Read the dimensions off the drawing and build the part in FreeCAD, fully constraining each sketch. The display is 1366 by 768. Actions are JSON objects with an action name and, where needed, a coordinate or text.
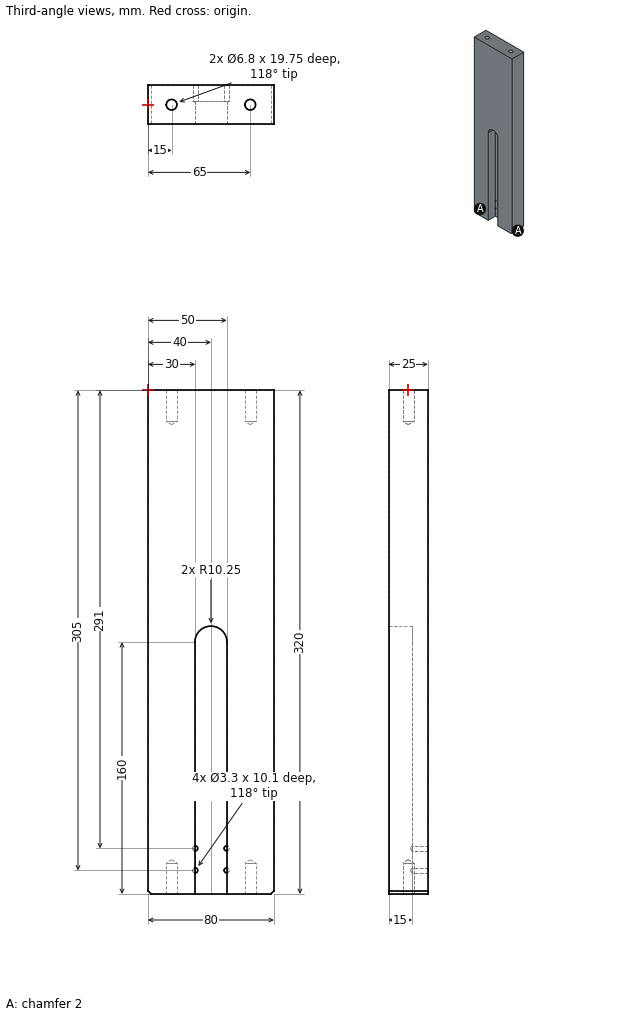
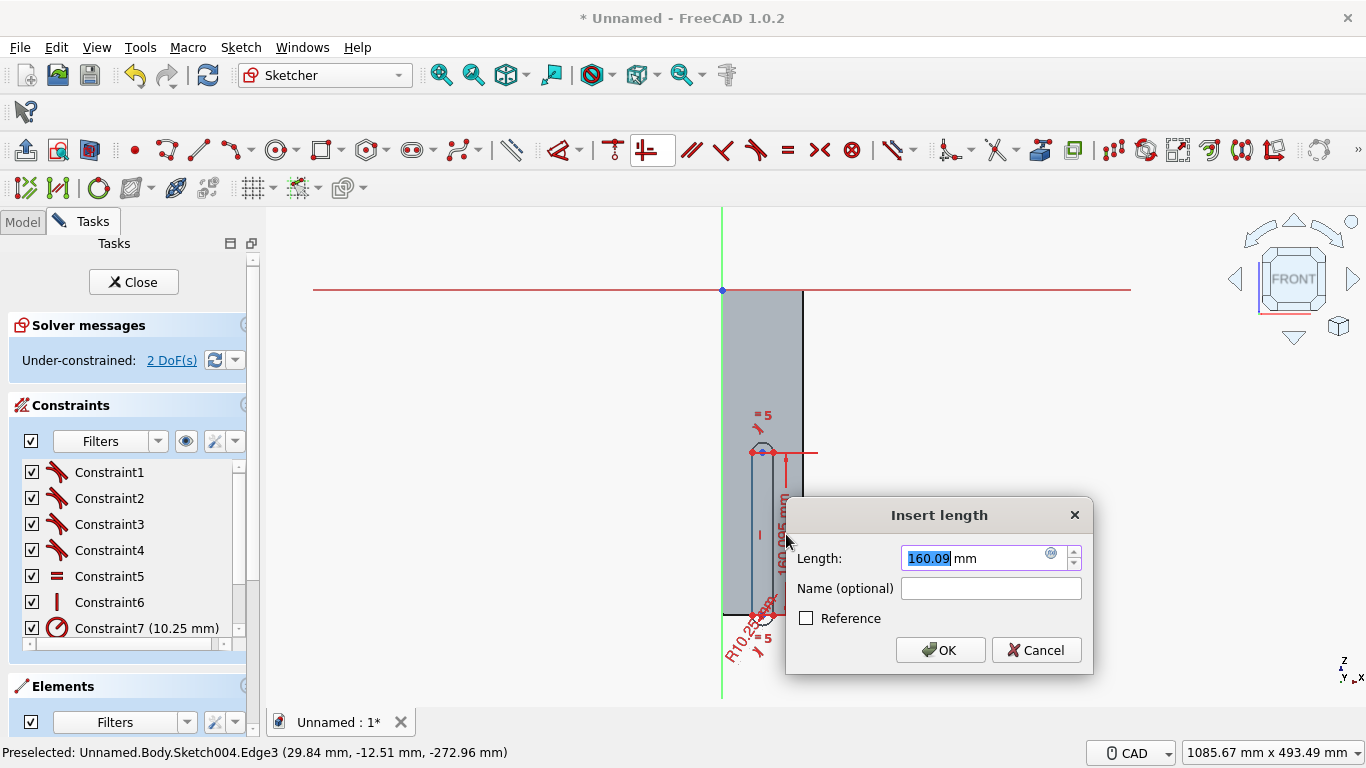
{"action": "type", "text": "160"}
{"action": "key", "text": "Return"}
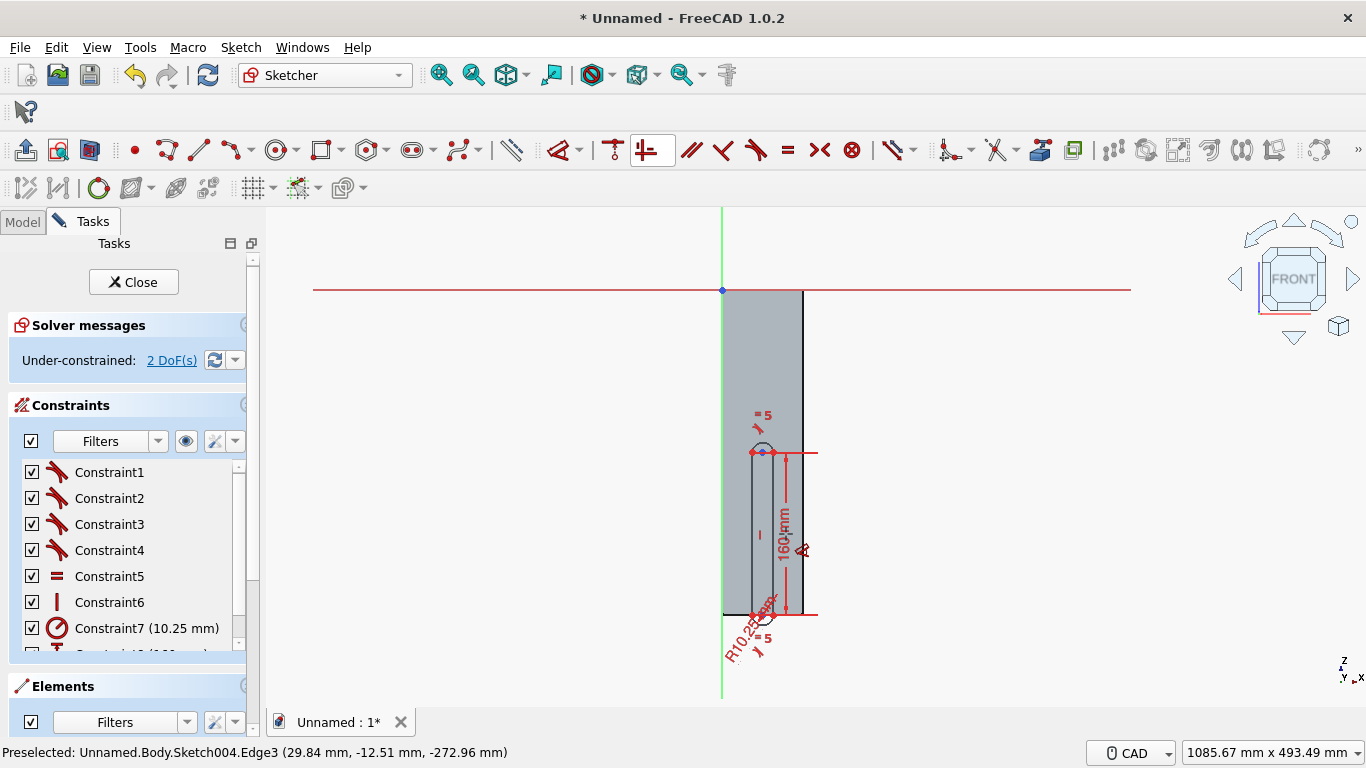
{"action": "left_click", "coordinate": [763, 615]}
{"action": "left_click", "coordinate": [743, 256]}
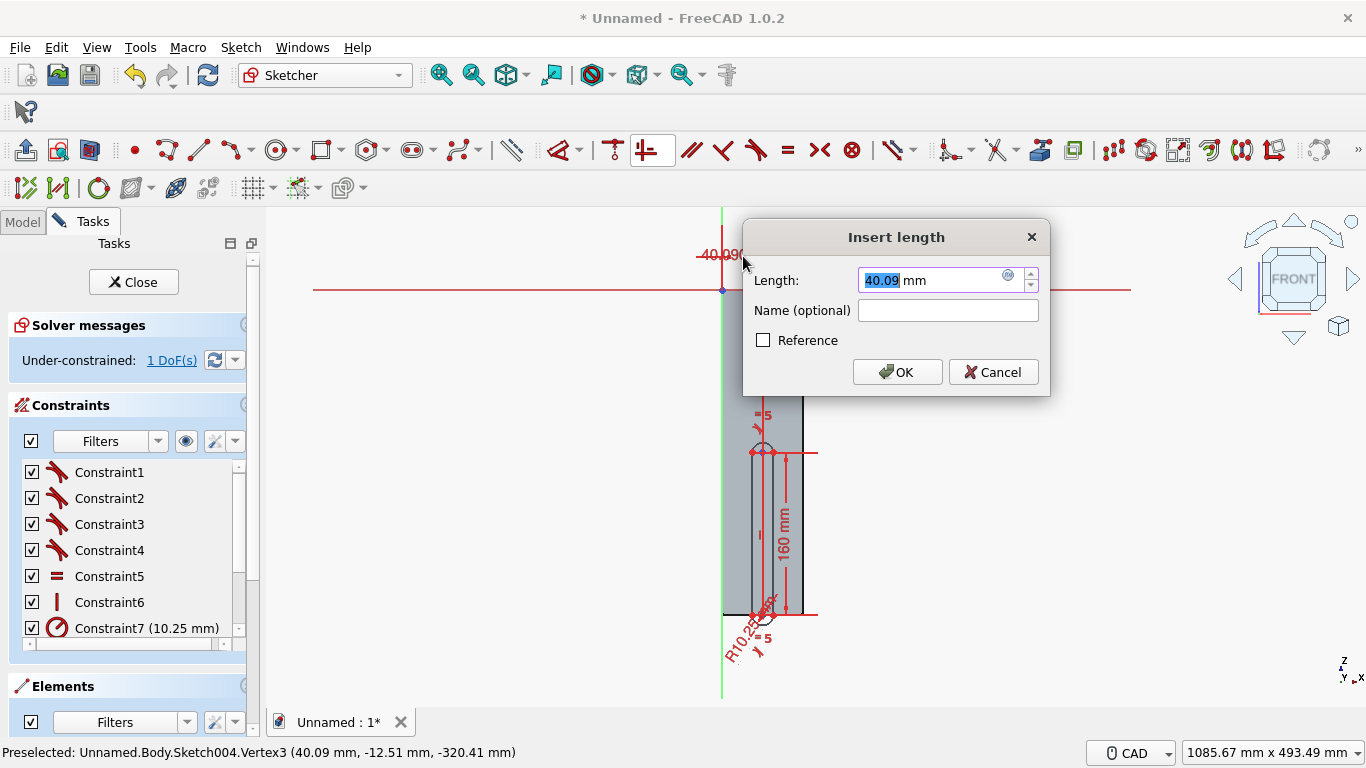
{"action": "type", "text": "40"}
{"action": "key", "text": "Return"}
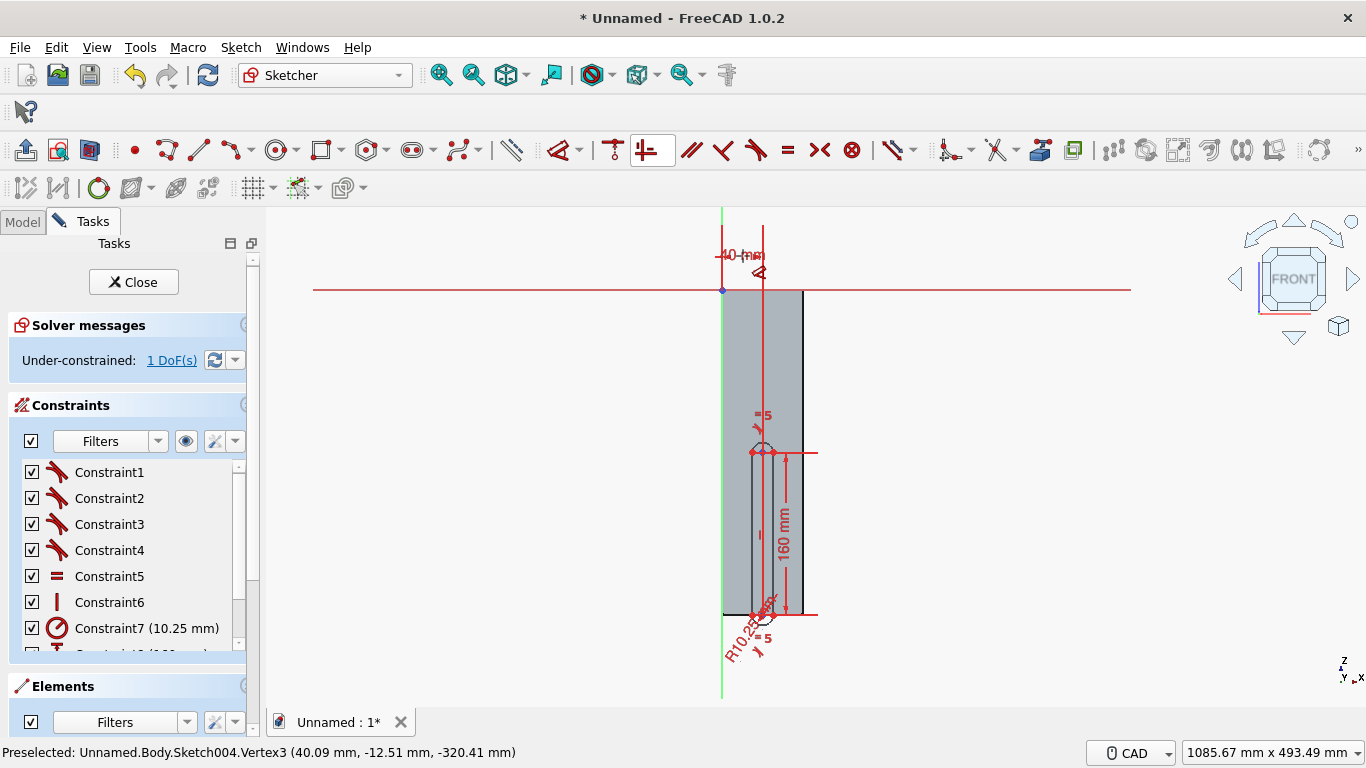
{"action": "left_click", "coordinate": [752, 615]}
{"action": "left_click", "coordinate": [688, 453]}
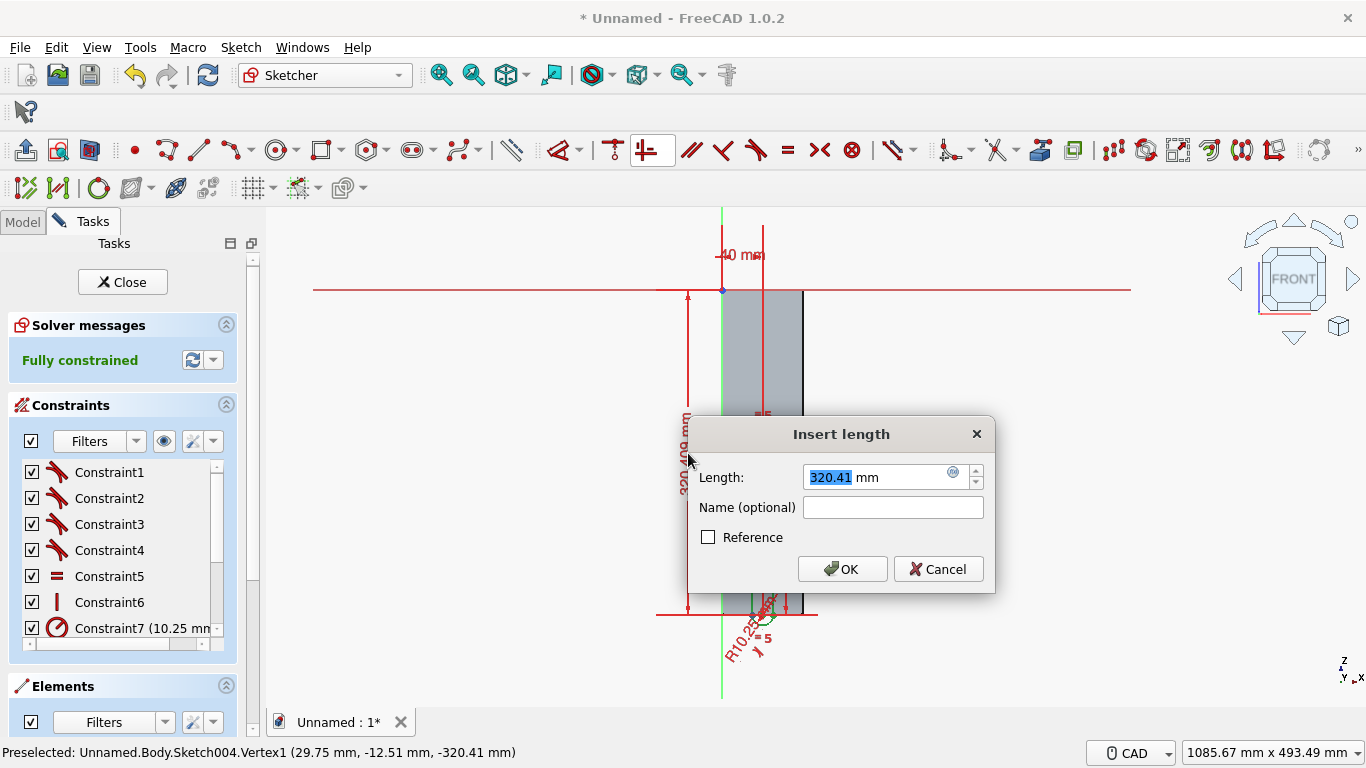
{"action": "type", "text": "320"}
{"action": "key", "text": "Return"}
{"action": "key", "text": "Escape"}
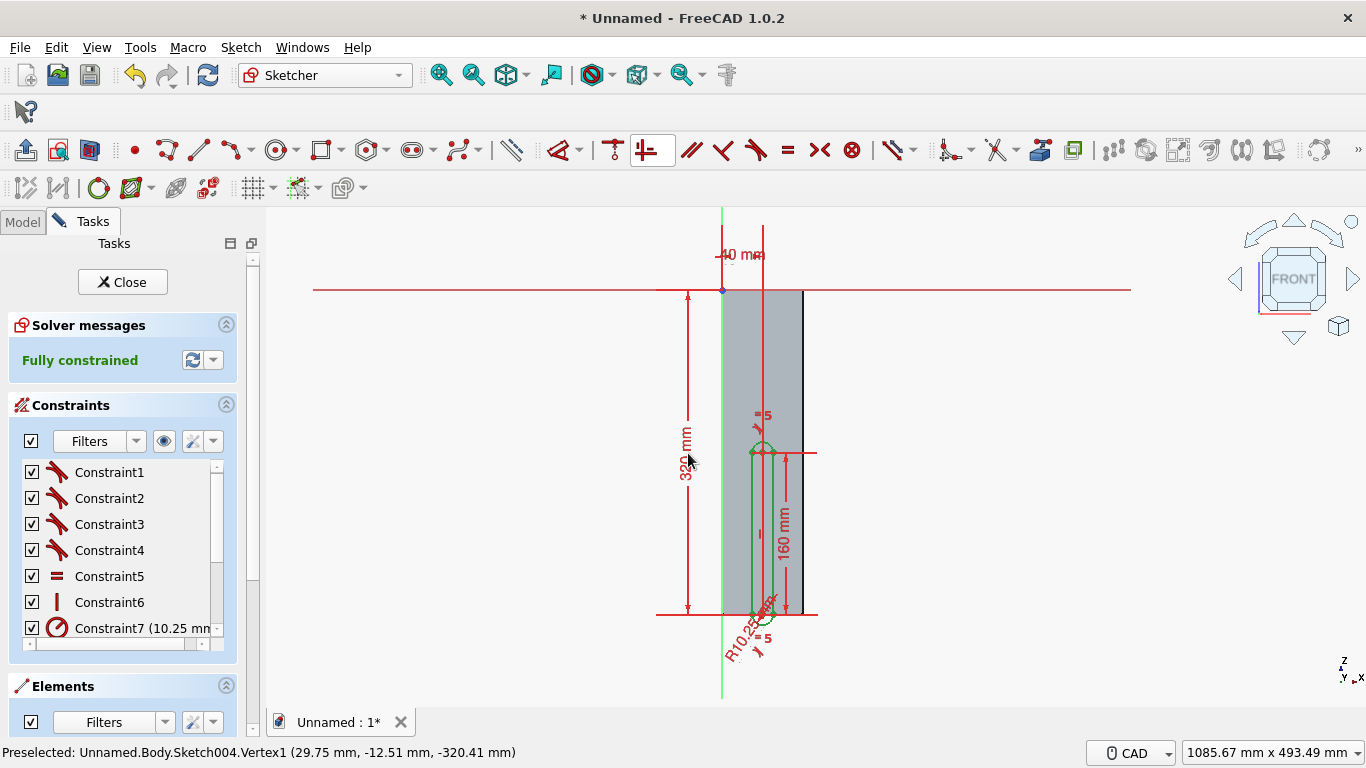
{"action": "left_click", "coordinate": [123, 282]}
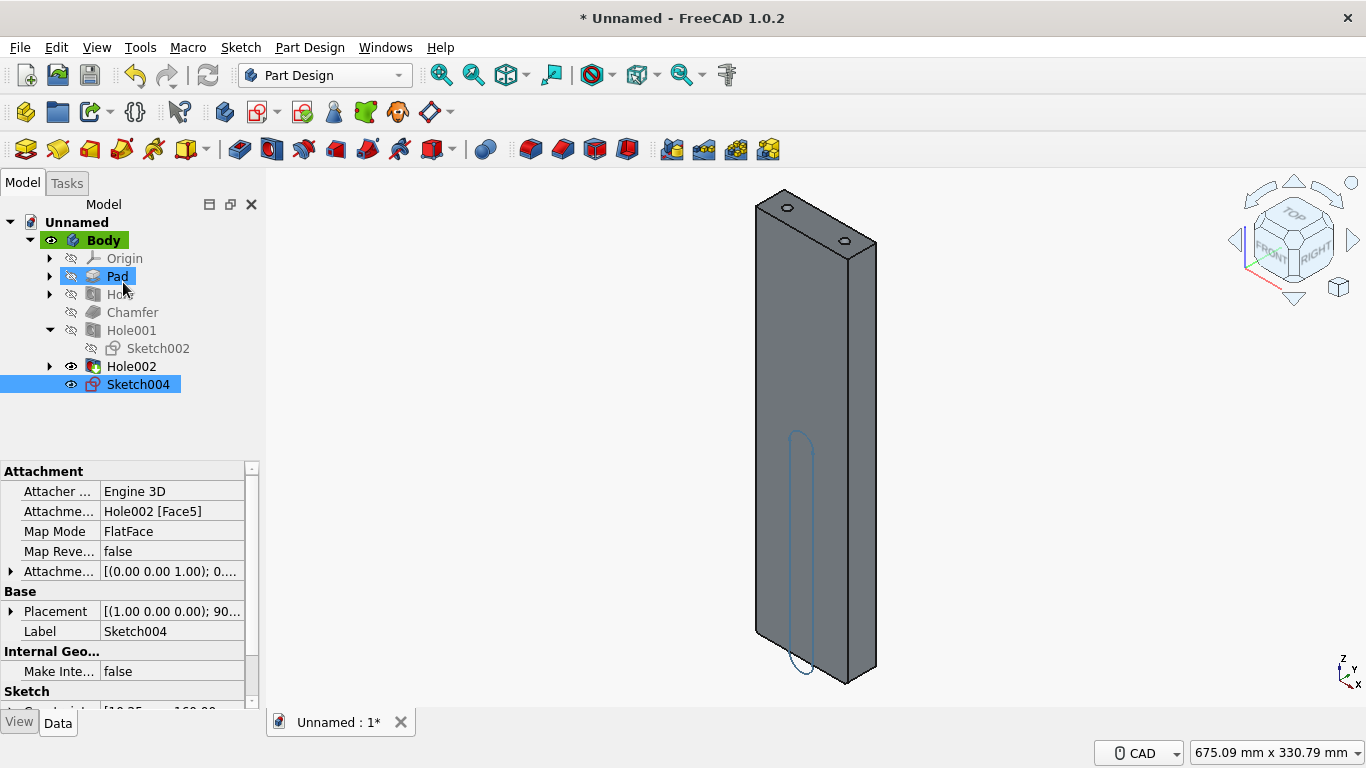
{"action": "left_click", "coordinate": [240, 150]}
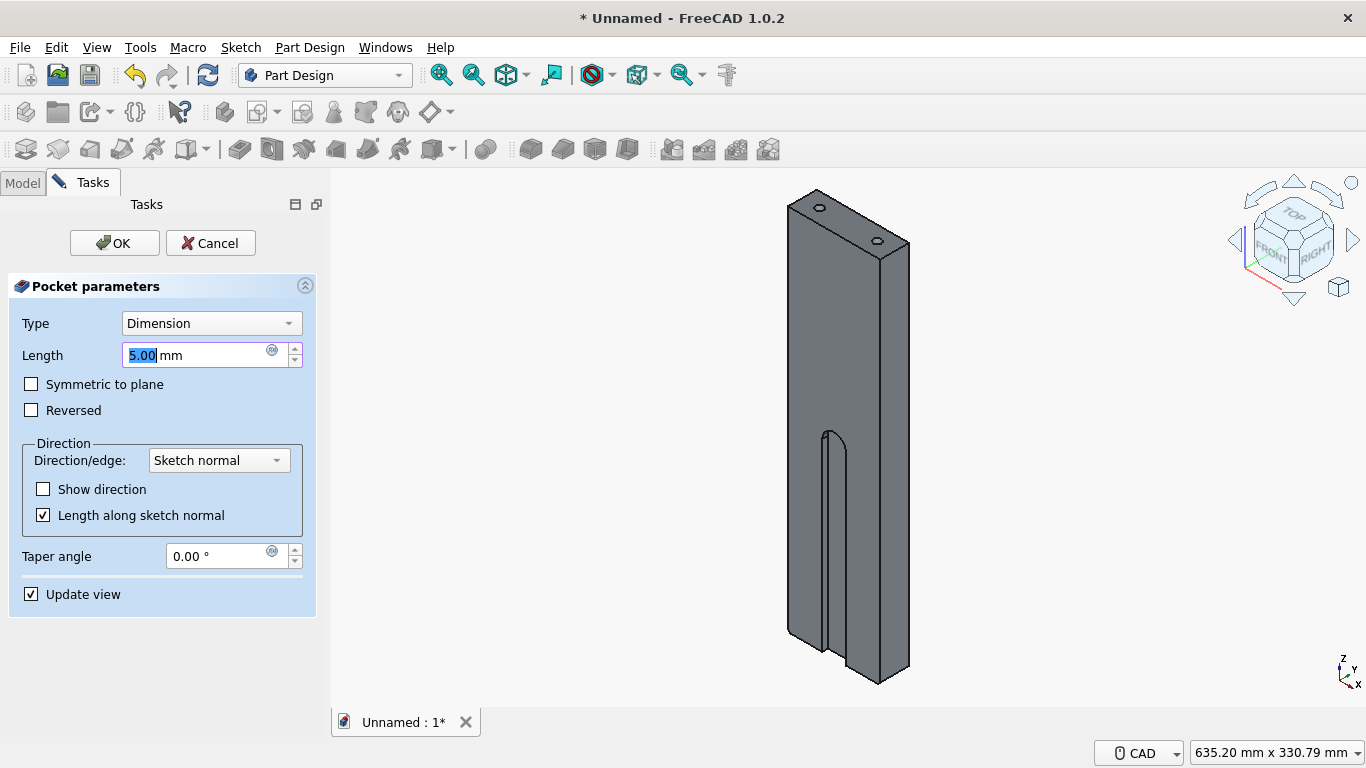
{"action": "type", "text": "15"}
{"action": "key", "text": "Tab"}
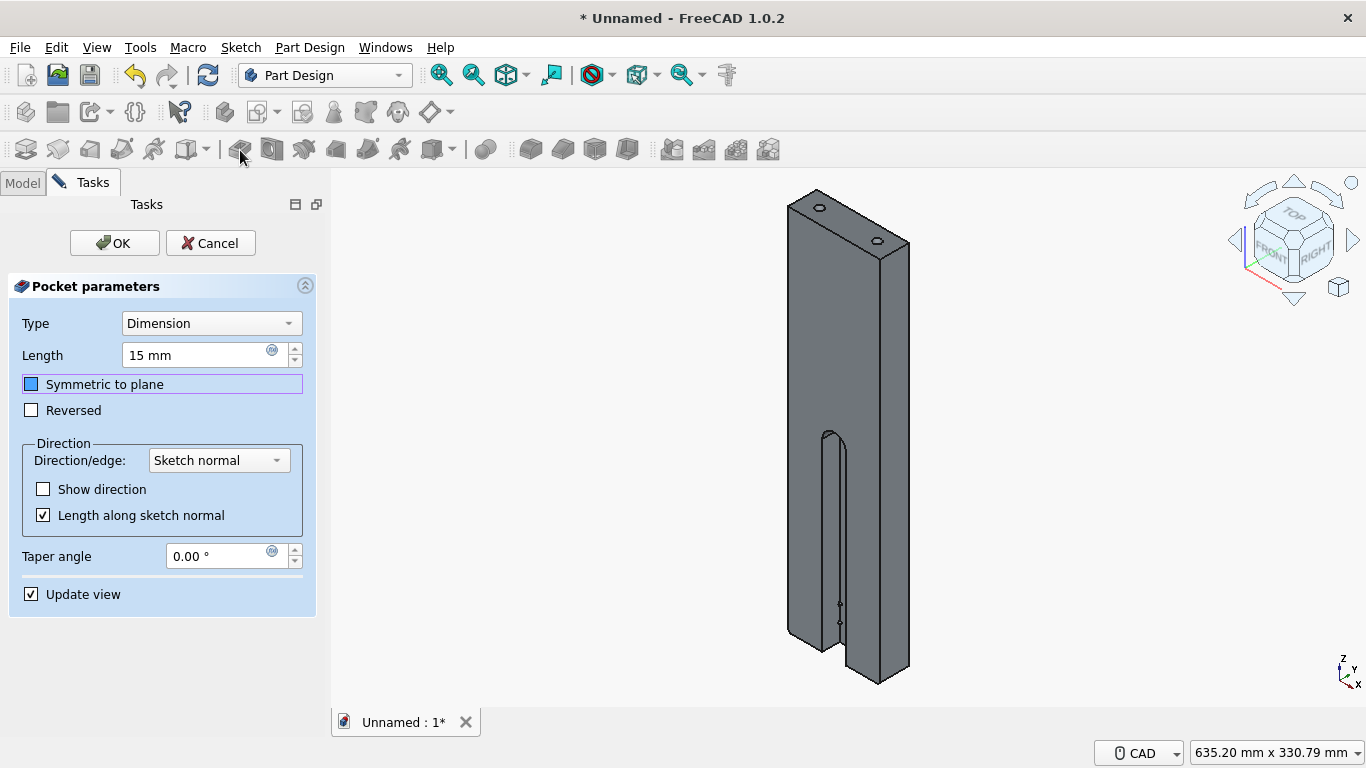
{"action": "left_click", "coordinate": [115, 243]}